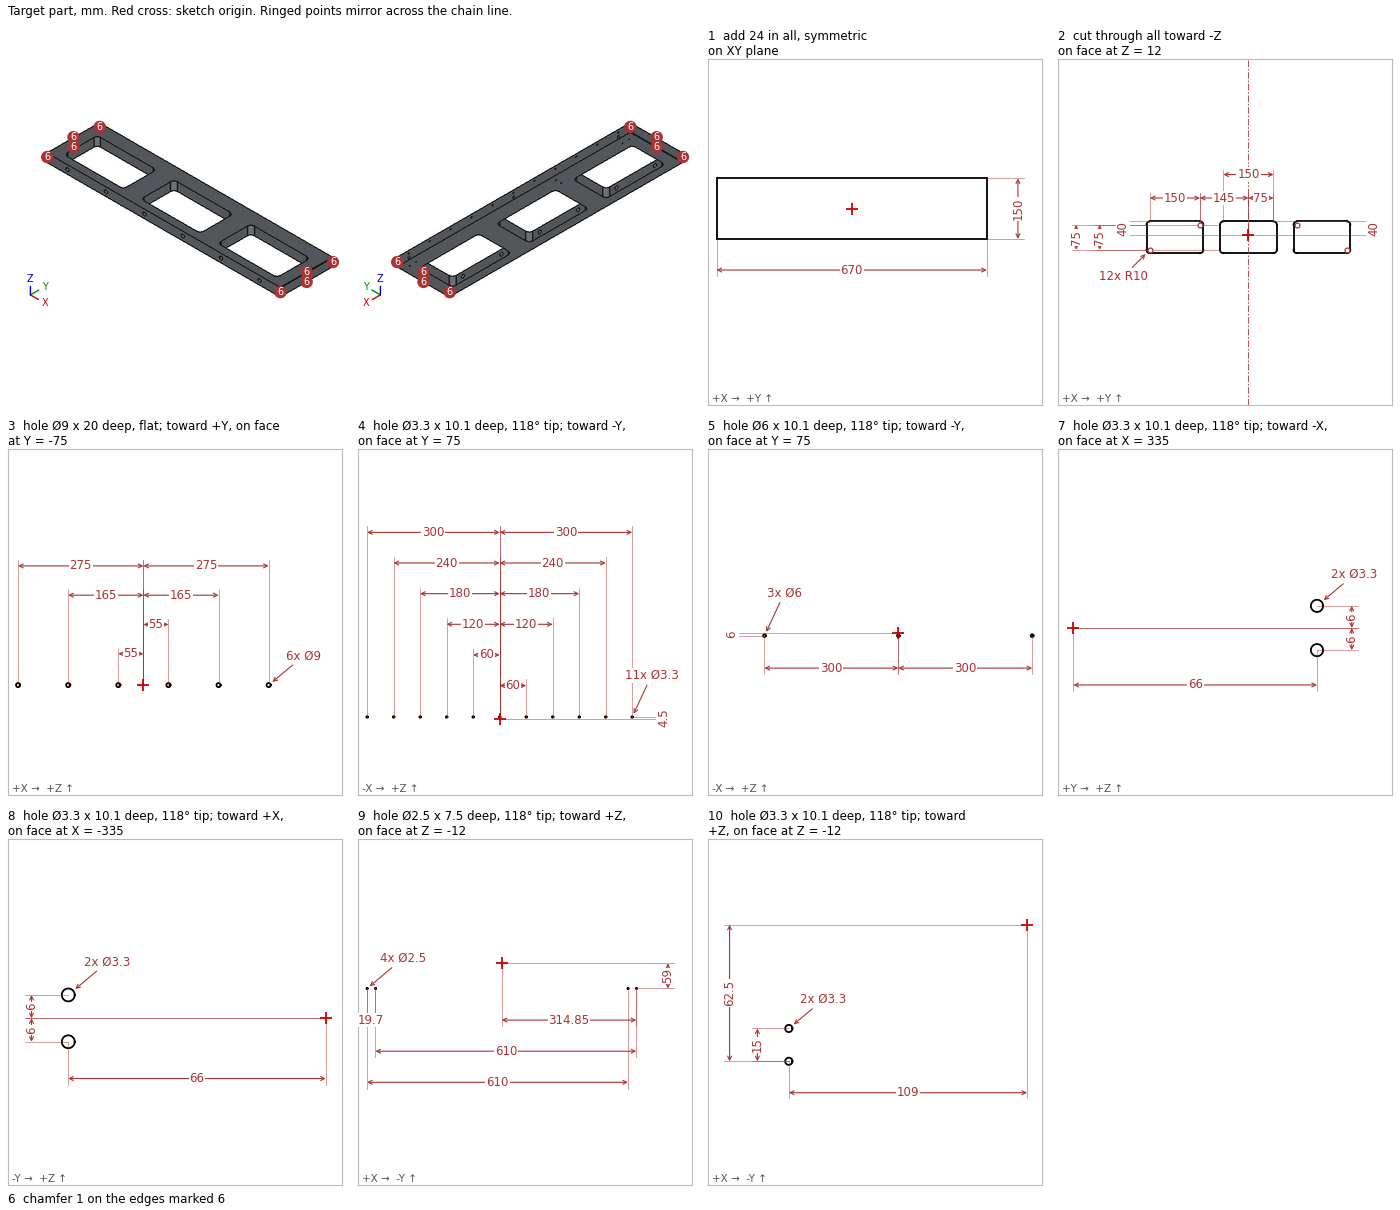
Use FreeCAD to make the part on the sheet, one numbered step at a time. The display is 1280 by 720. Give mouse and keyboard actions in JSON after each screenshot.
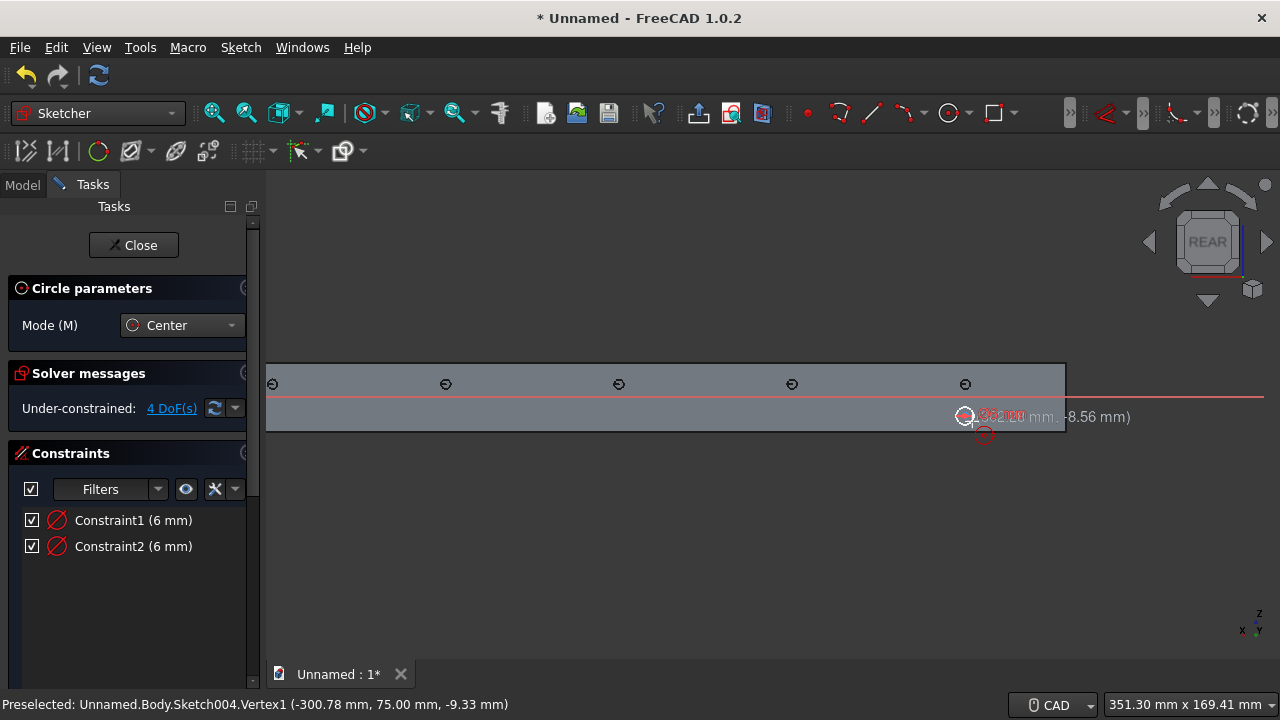
{"action": "scroll", "coordinate": [965, 416], "scroll_direction": "down", "scroll_amount": 6}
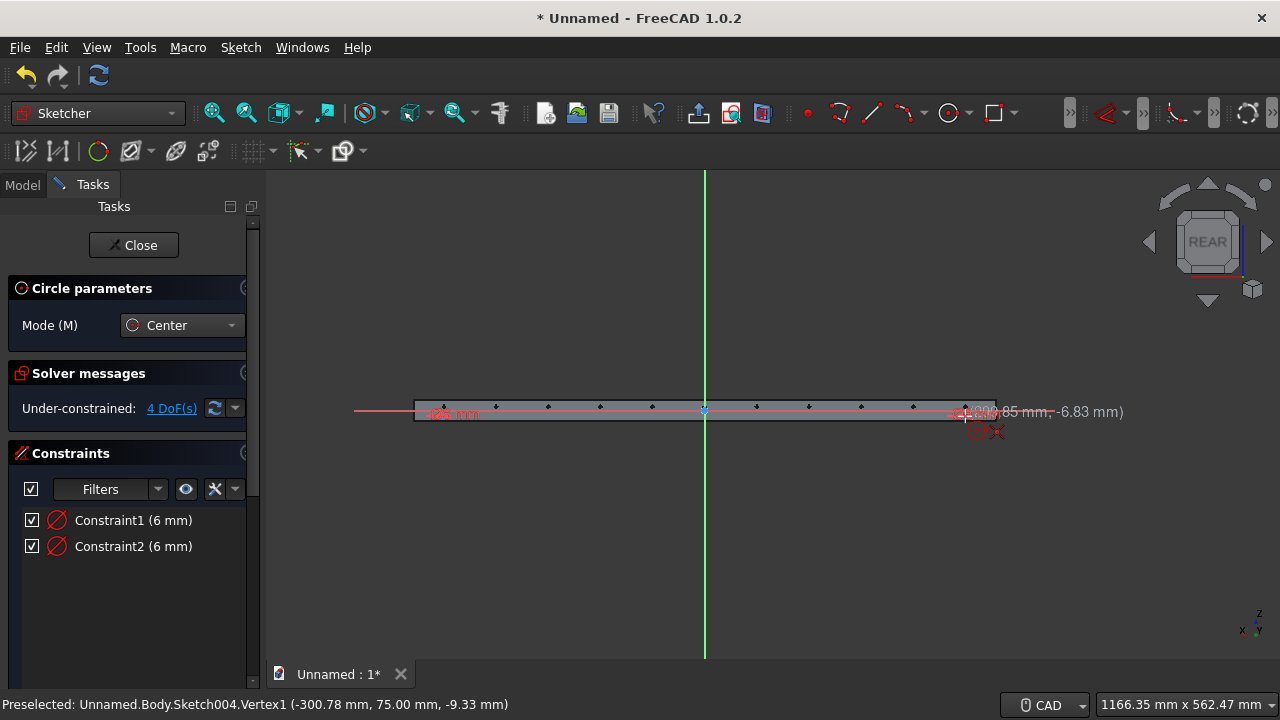
{"action": "scroll", "coordinate": [705, 416], "scroll_direction": "up", "scroll_amount": 11}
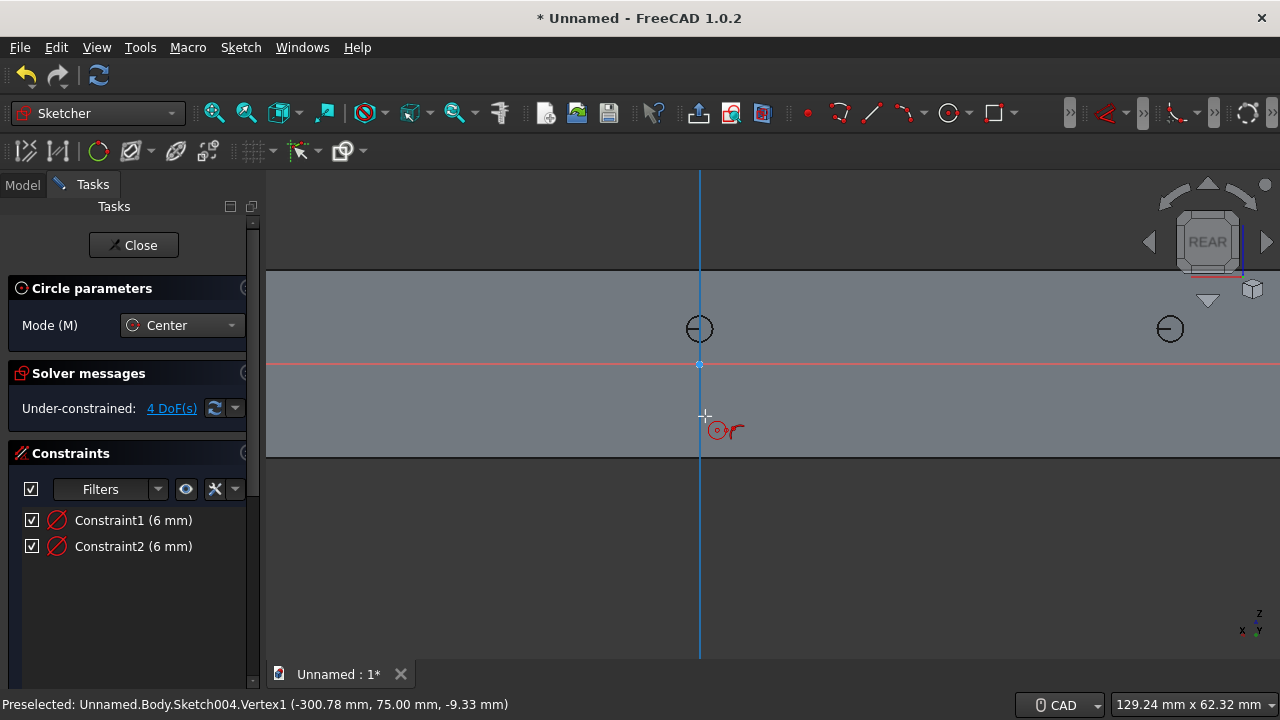
{"action": "scroll", "coordinate": [705, 416], "scroll_direction": "down", "scroll_amount": 11}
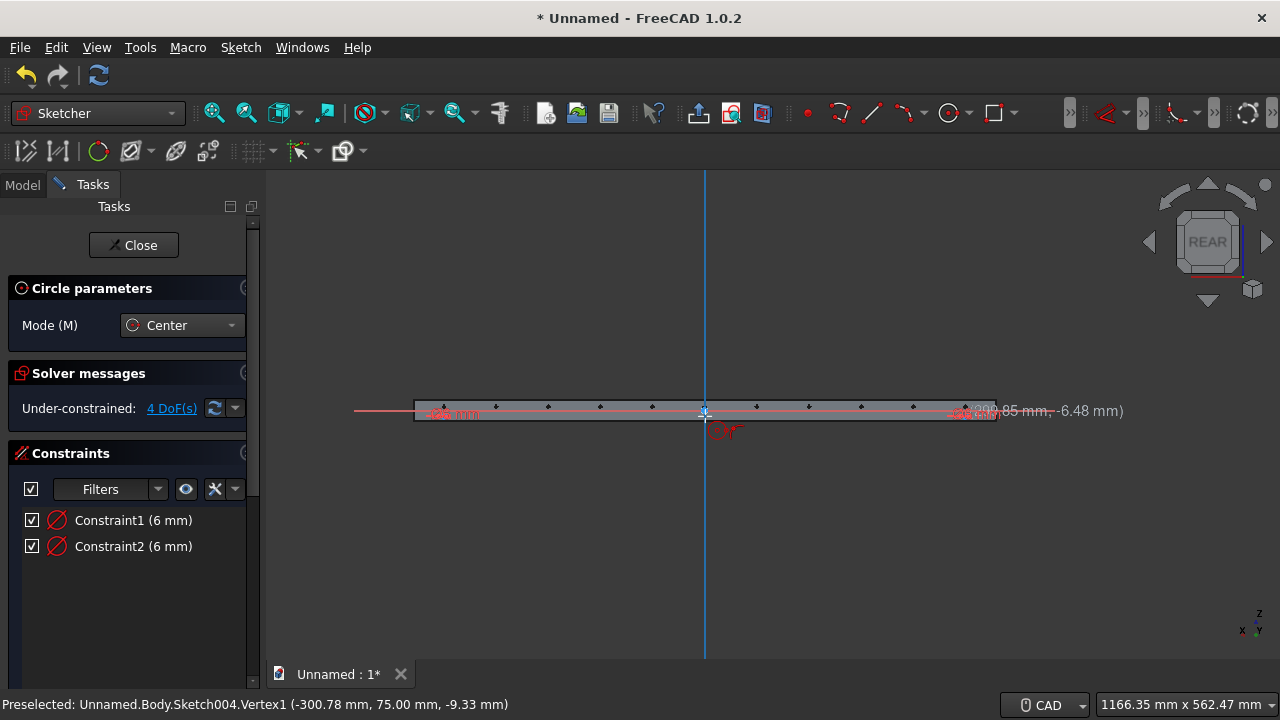
{"action": "scroll", "coordinate": [705, 416], "scroll_direction": "up", "scroll_amount": 6}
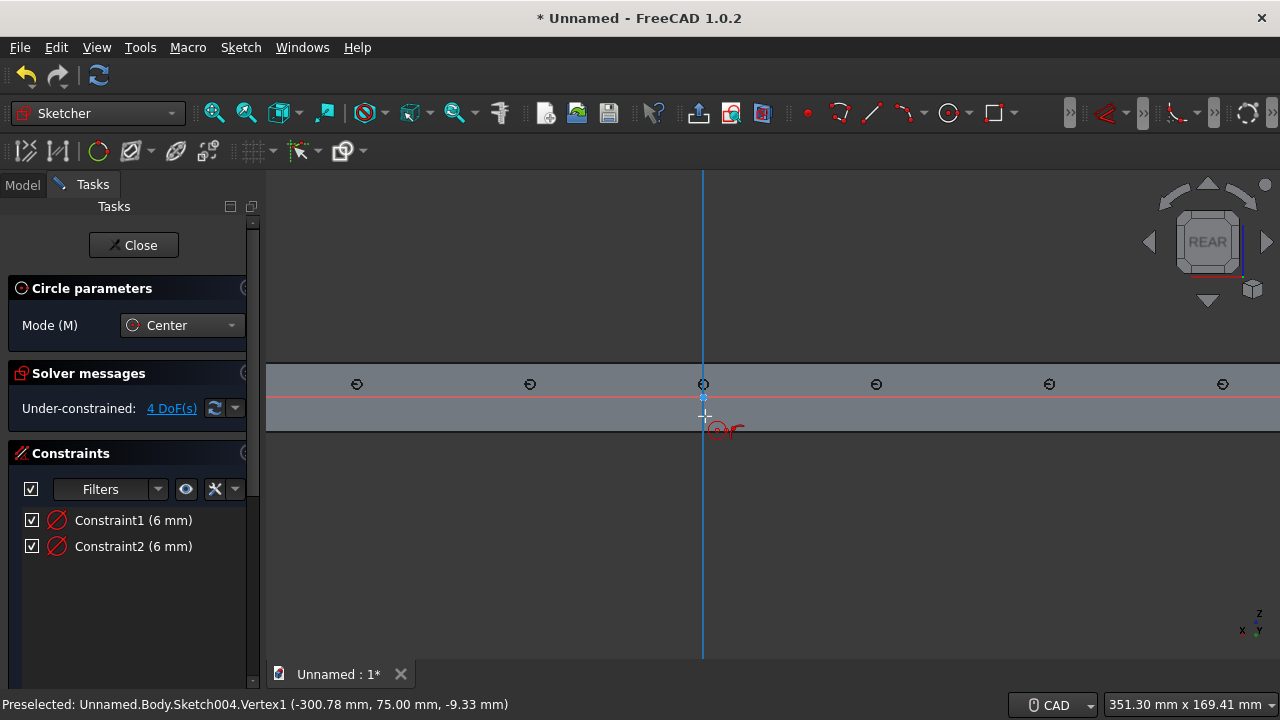
{"action": "left_click", "coordinate": [703, 415]}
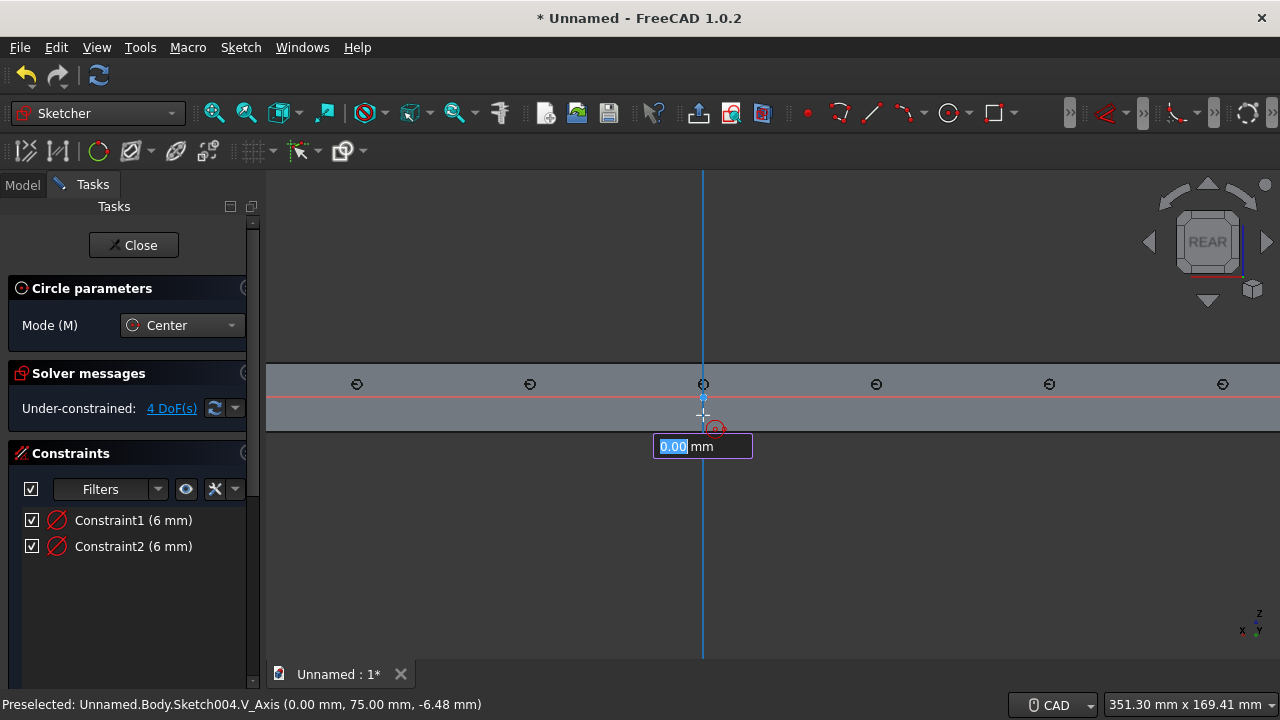
{"action": "scroll", "coordinate": [711, 412], "scroll_direction": "up", "scroll_amount": 4}
{"action": "mouse_move", "coordinate": [711, 411]}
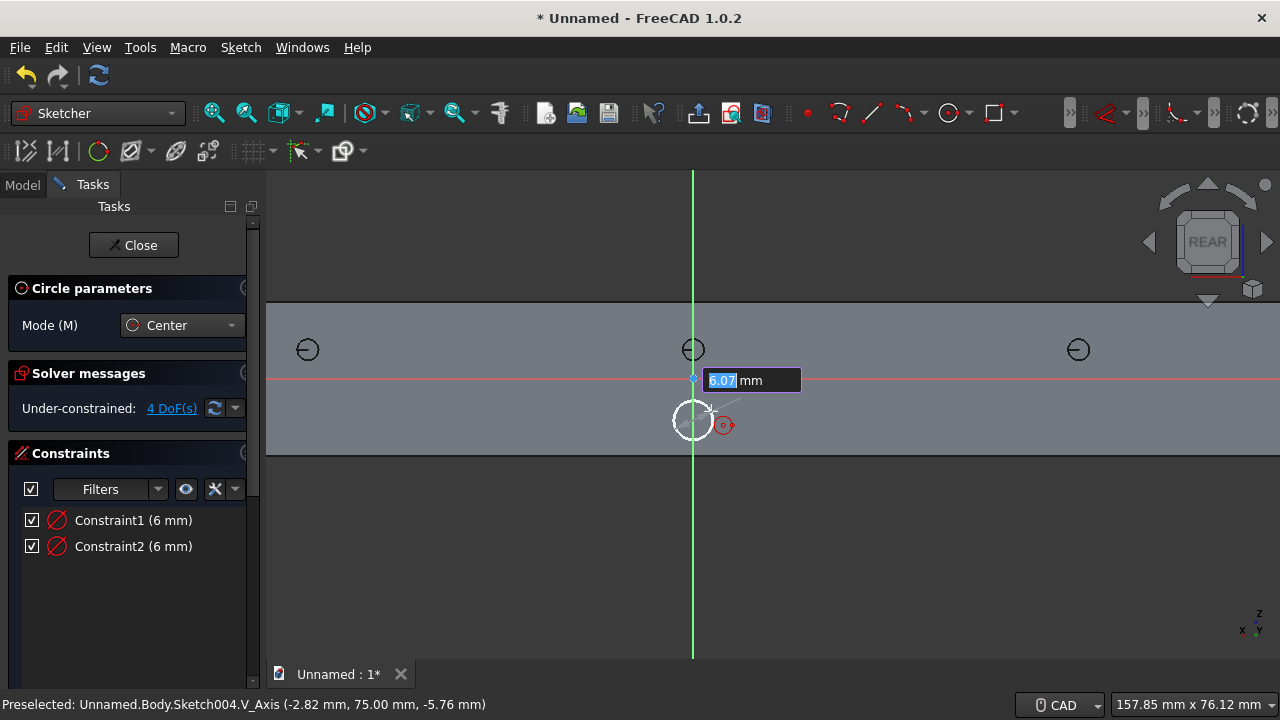
{"action": "type", "text": "6"}
{"action": "key", "text": "Return"}
{"action": "key", "text": "Escape"}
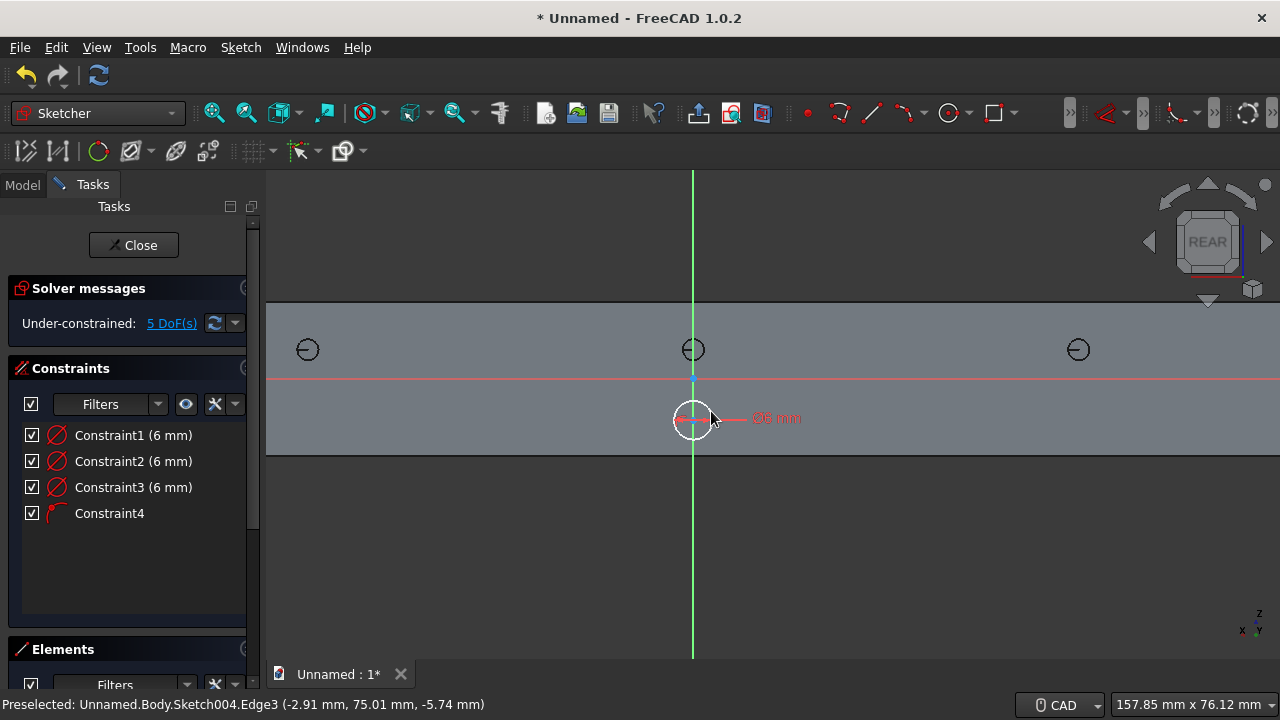
{"action": "scroll", "coordinate": [706, 416], "scroll_direction": "down", "scroll_amount": 10}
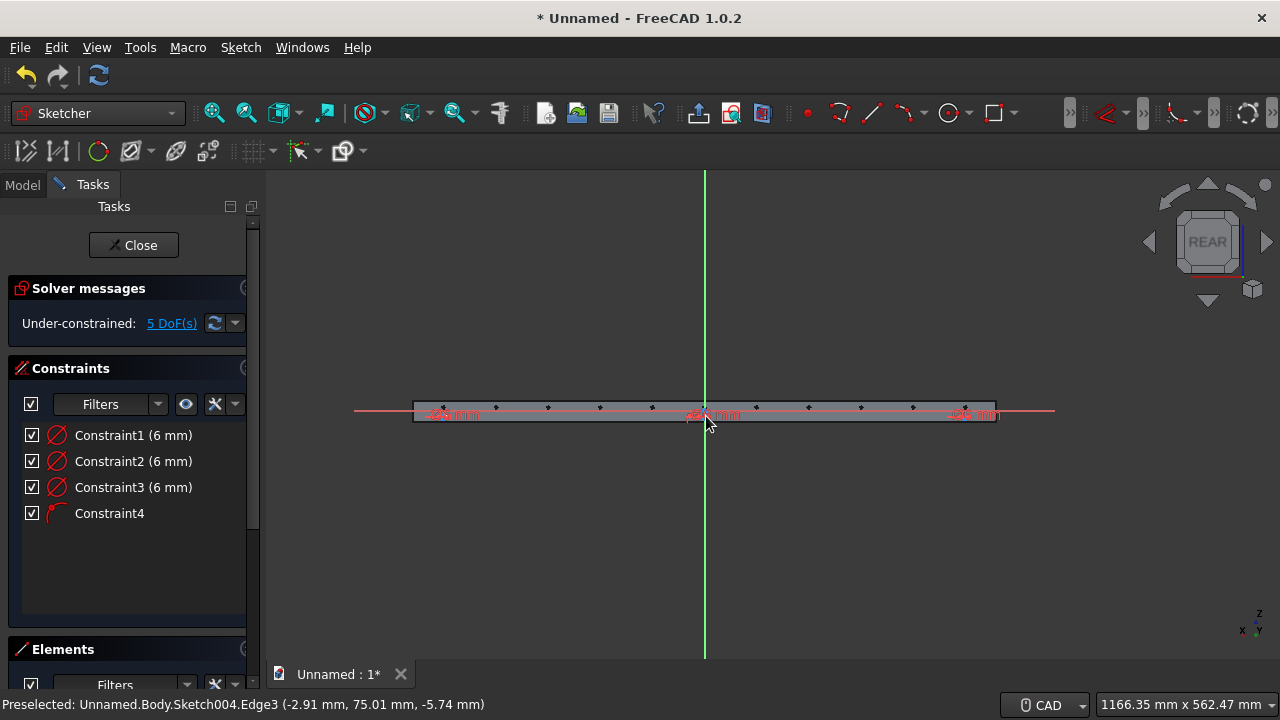
{"action": "left_click", "coordinate": [444, 417]}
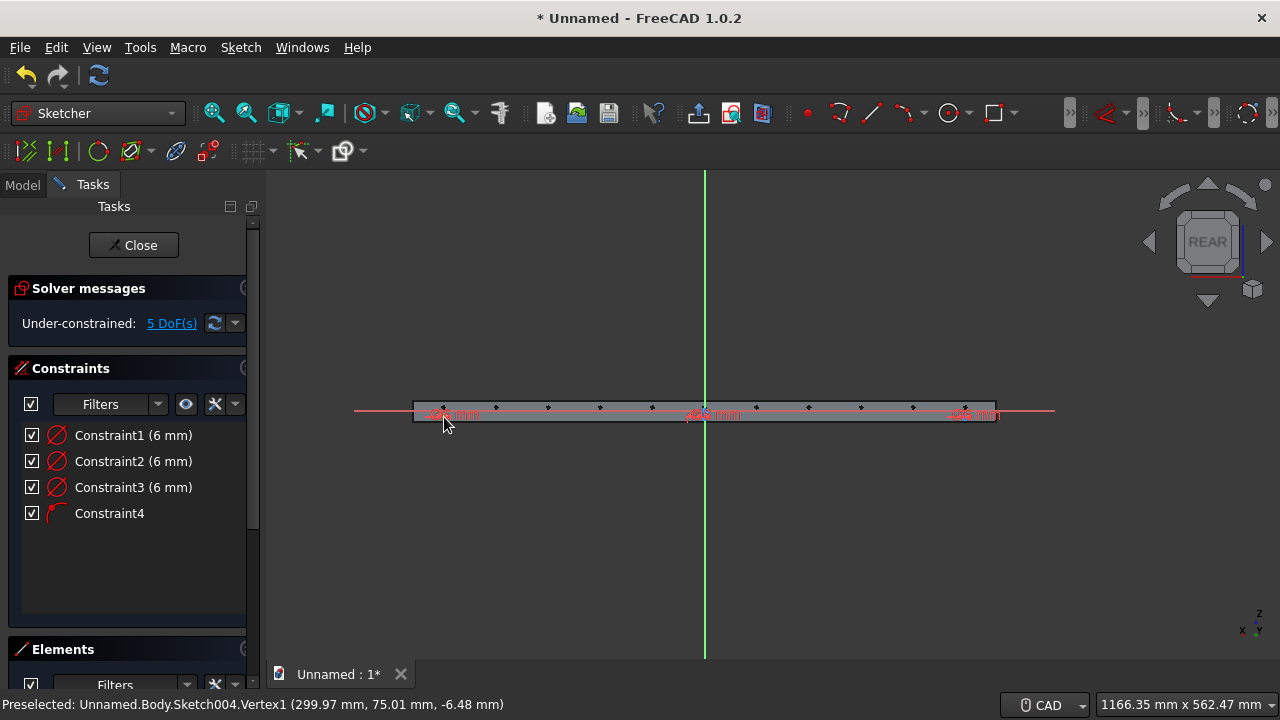
{"action": "left_click", "coordinate": [965, 417]}